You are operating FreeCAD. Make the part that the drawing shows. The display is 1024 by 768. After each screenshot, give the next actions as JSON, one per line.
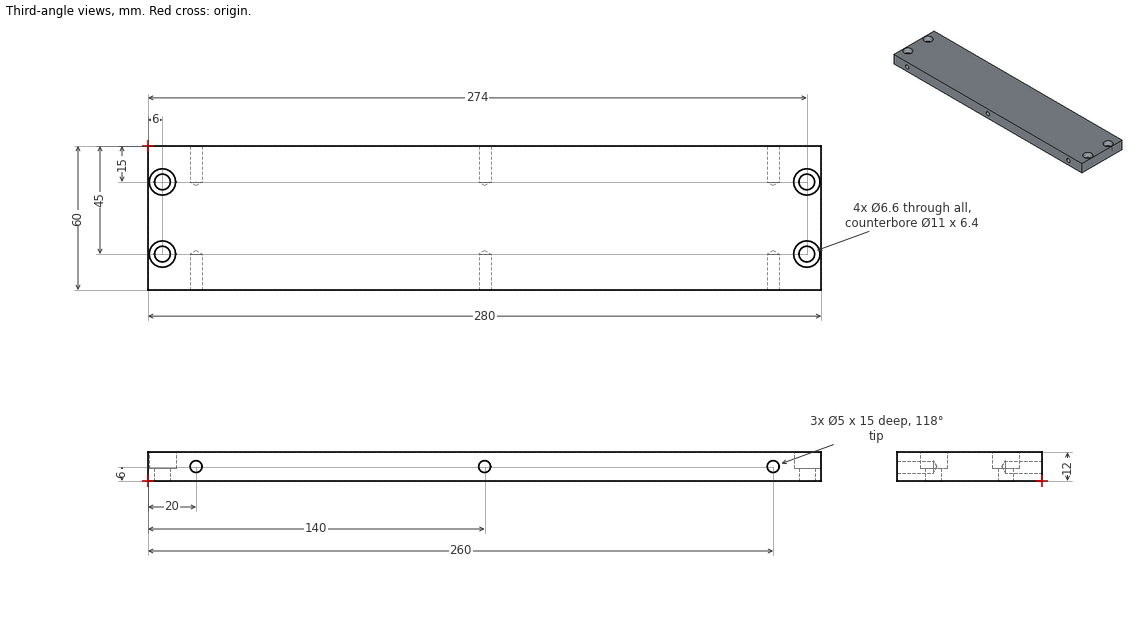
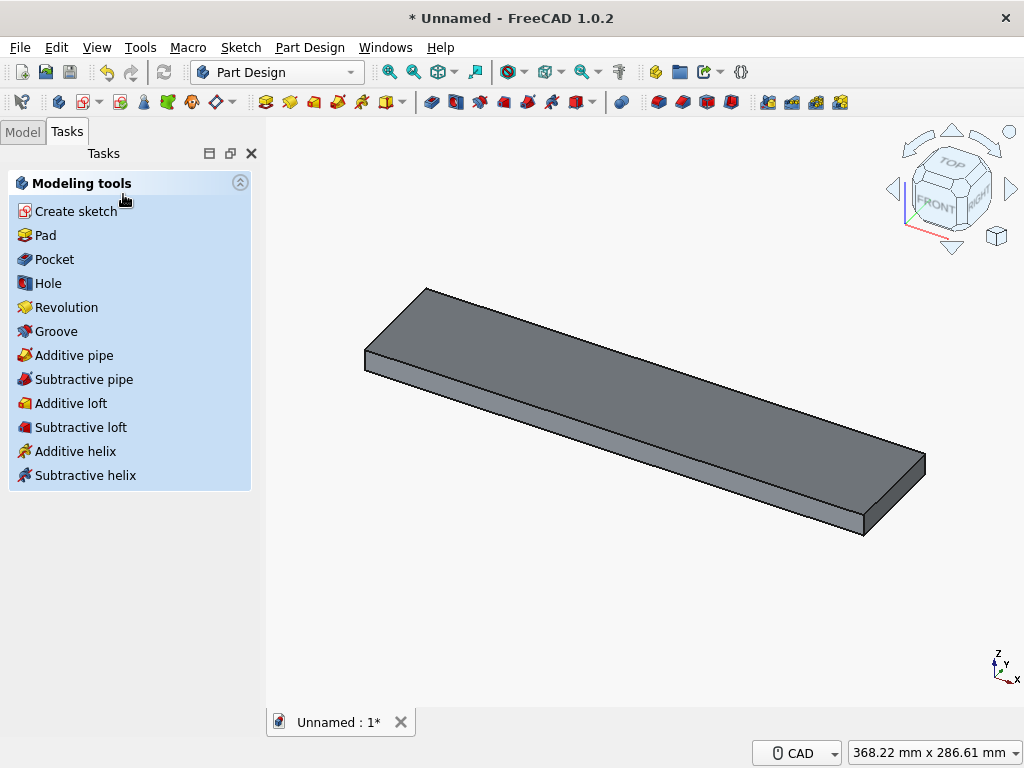
{"action": "left_click", "coordinate": [456, 102]}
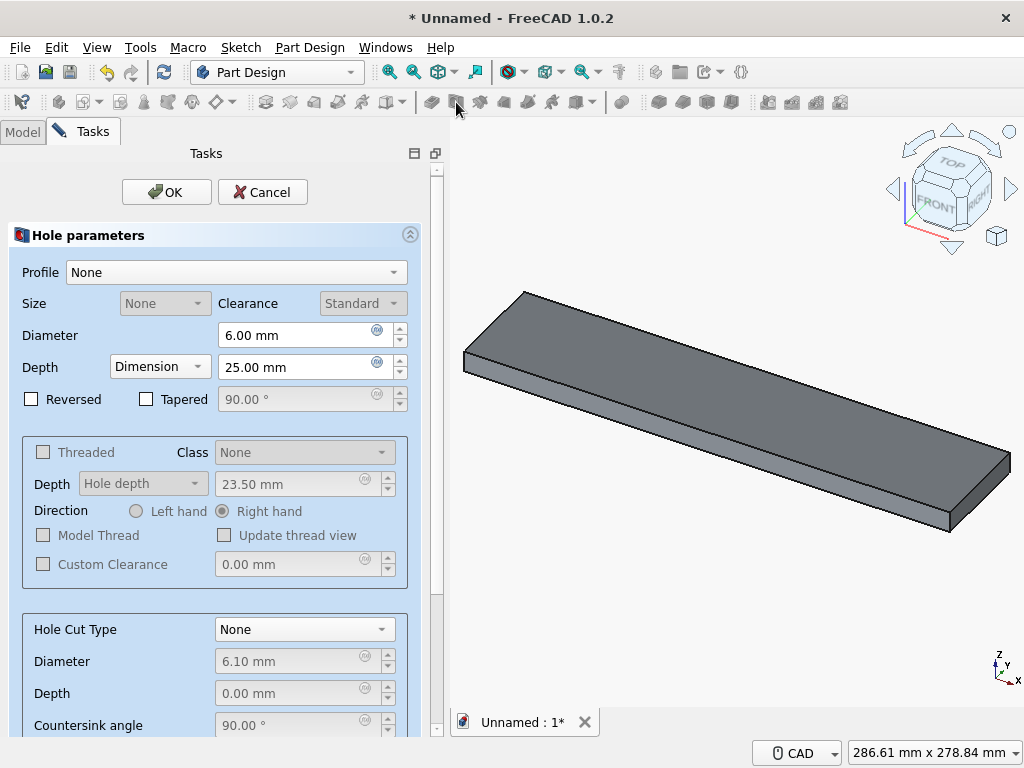
{"action": "triple_click", "coordinate": [305, 335]}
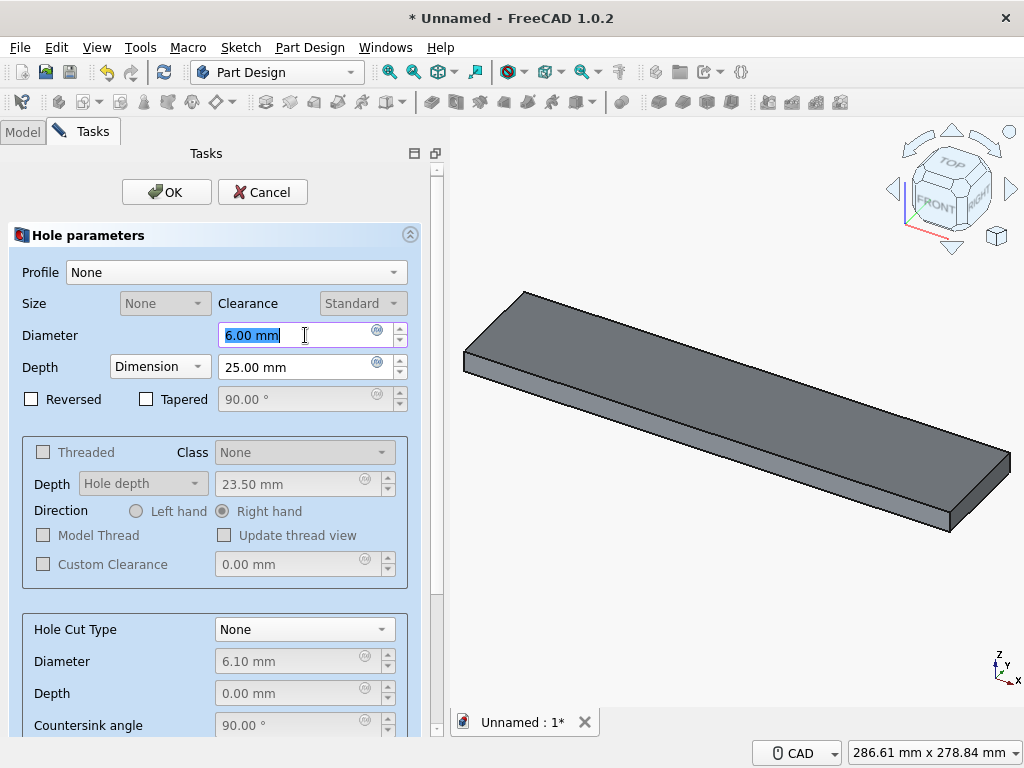
{"action": "type", "text": "5"}
{"action": "key", "text": "Tab"}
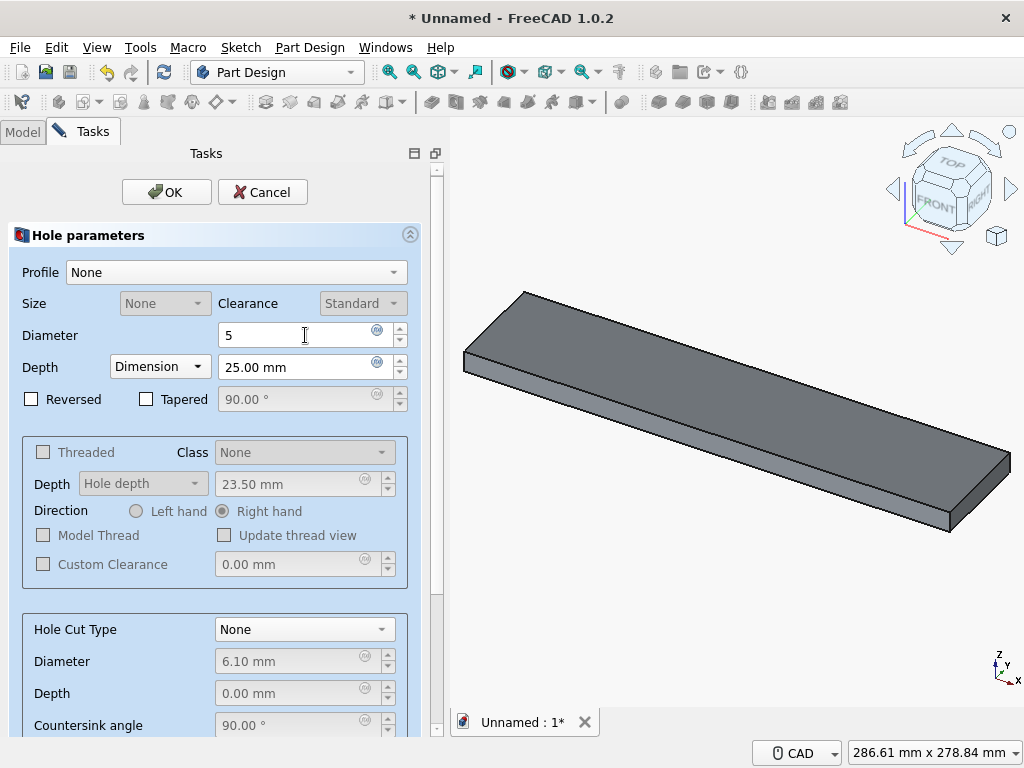
{"action": "triple_click", "coordinate": [305, 367]}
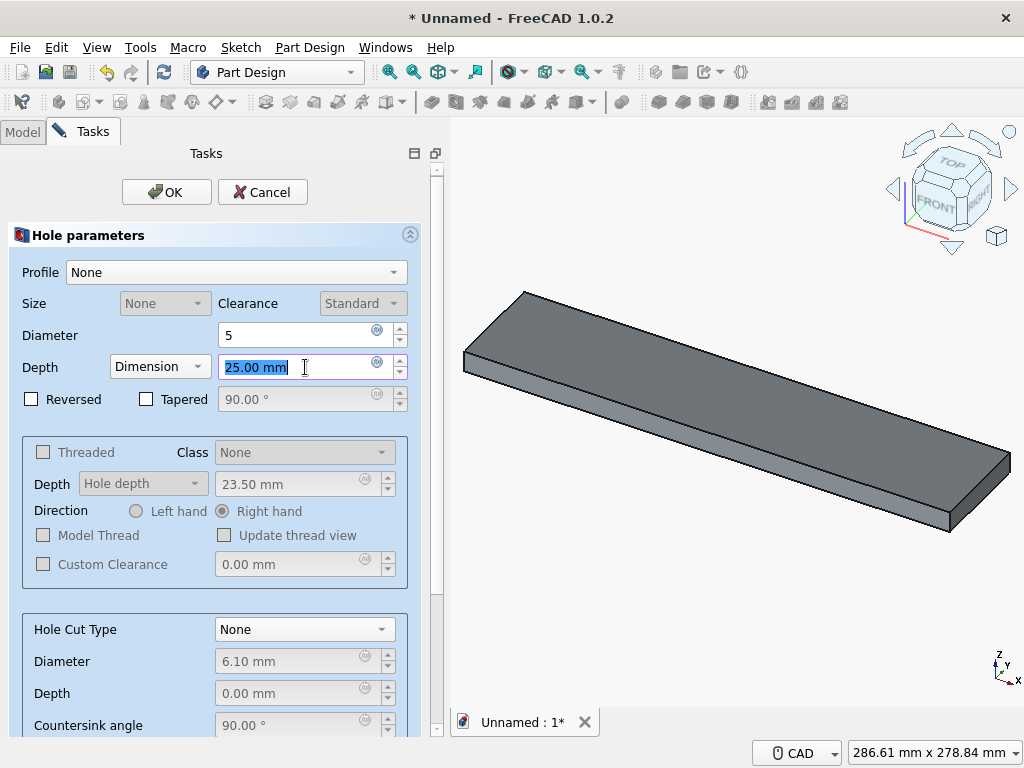
{"action": "type", "text": "15"}
{"action": "key", "text": "Tab"}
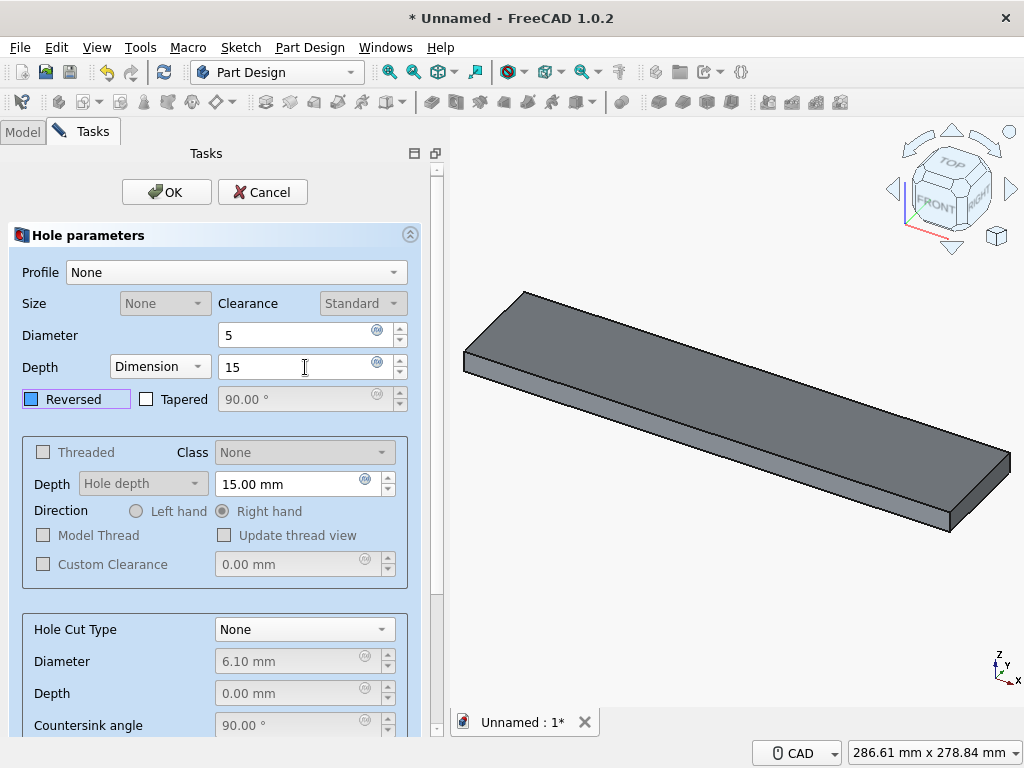
{"action": "left_click", "coordinate": [30, 399]}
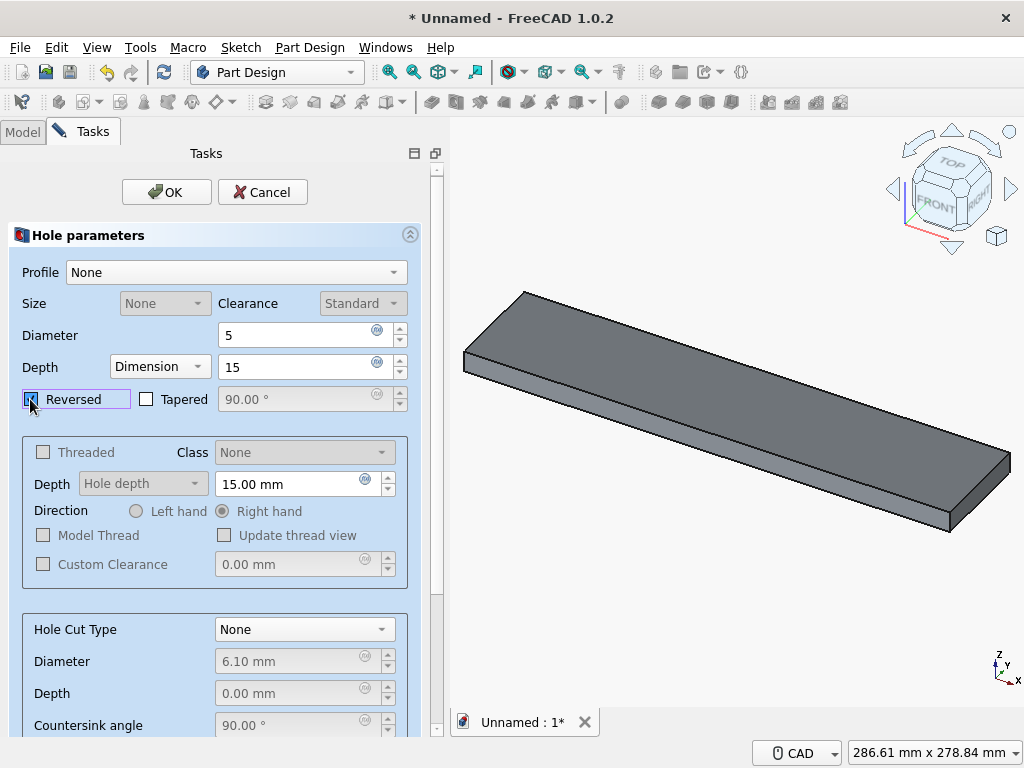
{"action": "left_click", "coordinate": [167, 192]}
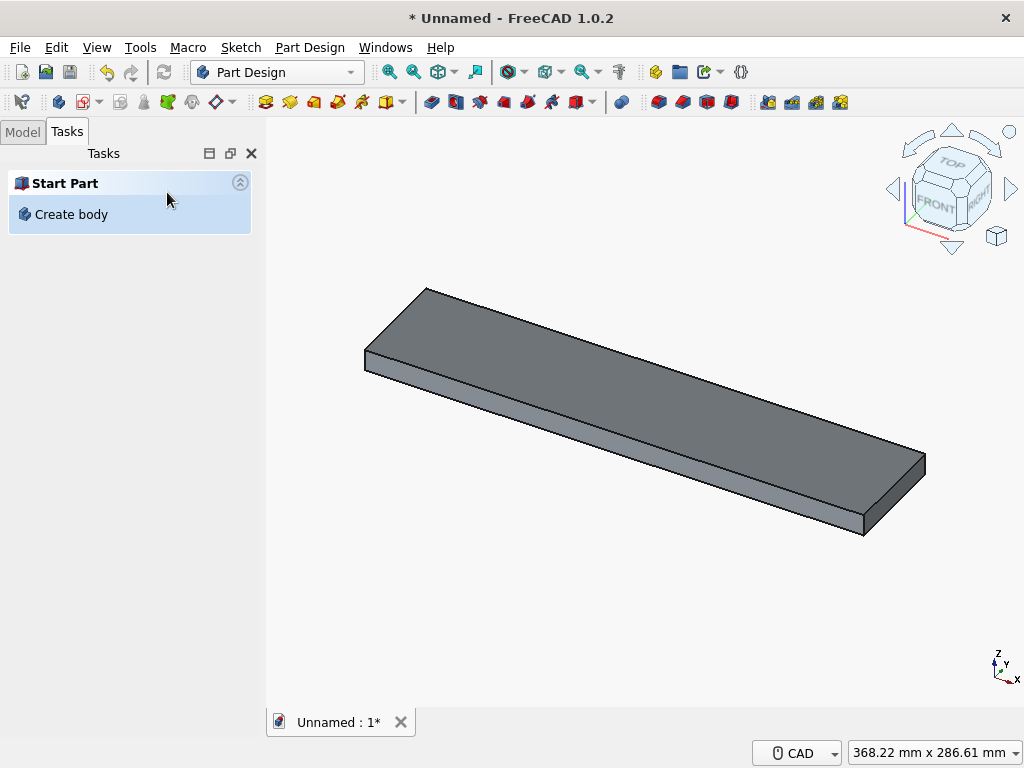
{"action": "left_click", "coordinate": [828, 513]}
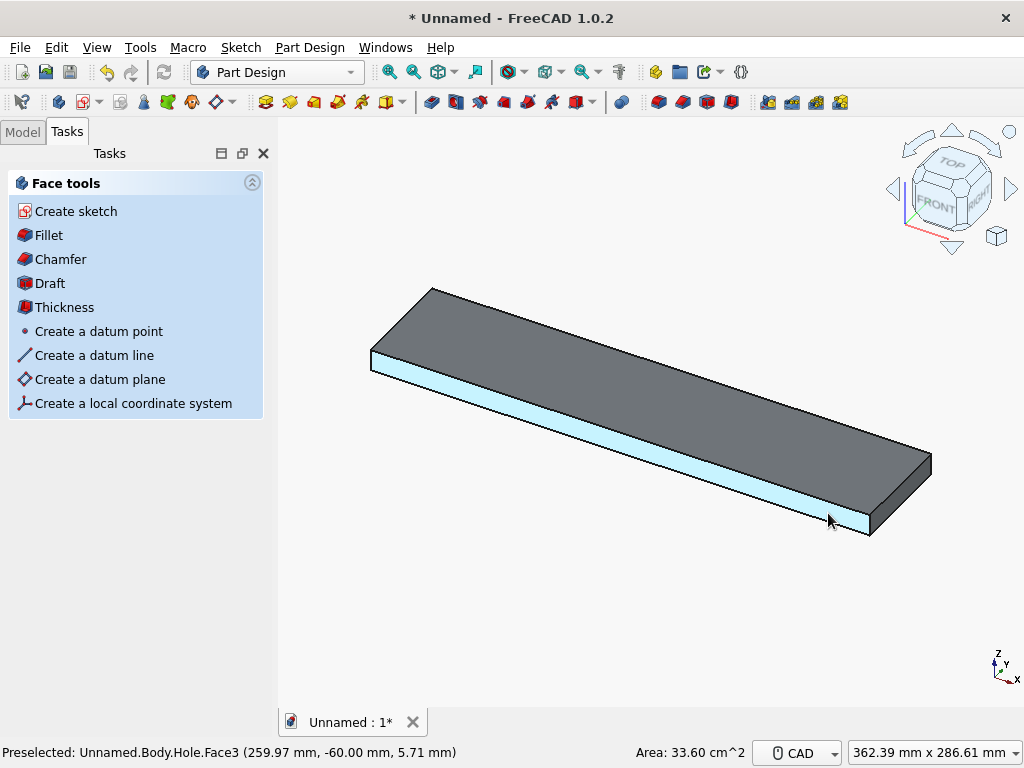
{"action": "left_click", "coordinate": [84, 102]}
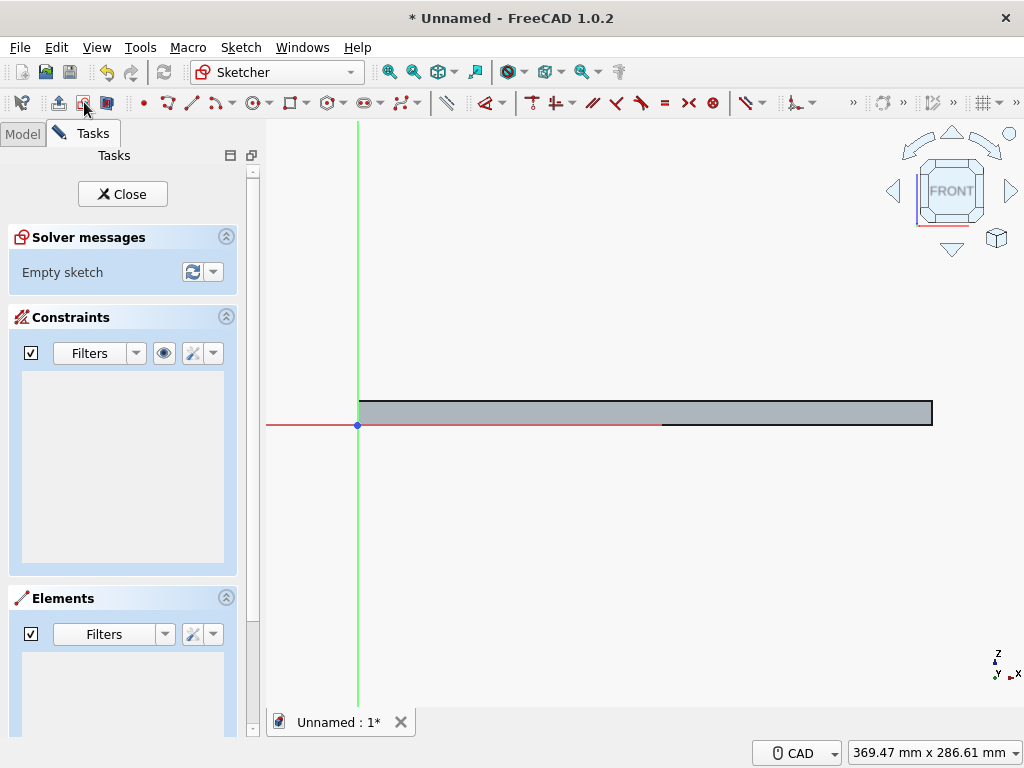
{"action": "scroll", "coordinate": [474, 406], "scroll_direction": "down", "scroll_amount": 2}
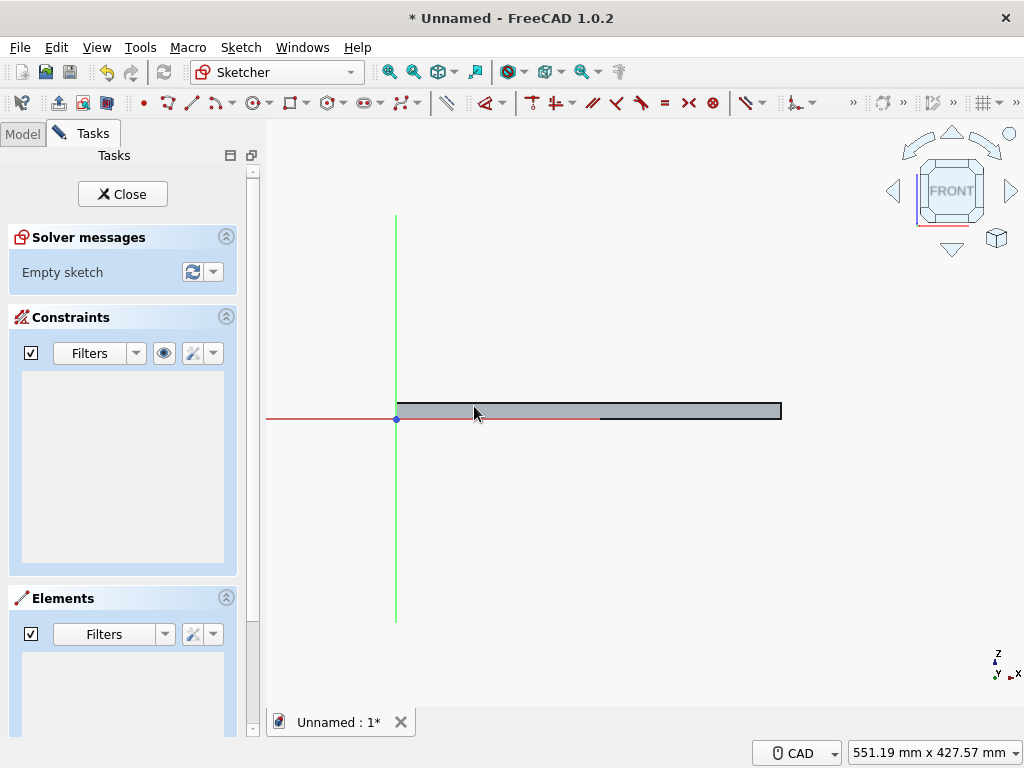
{"action": "left_click", "coordinate": [254, 104]}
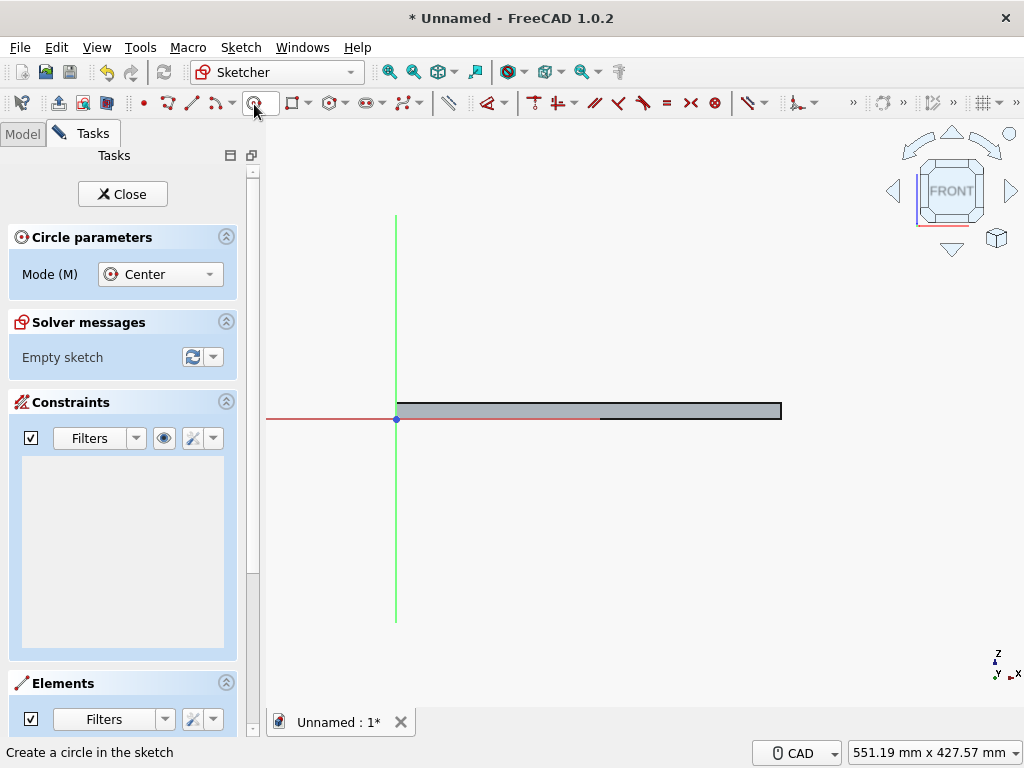
{"action": "scroll", "coordinate": [754, 411], "scroll_direction": "up", "scroll_amount": 10}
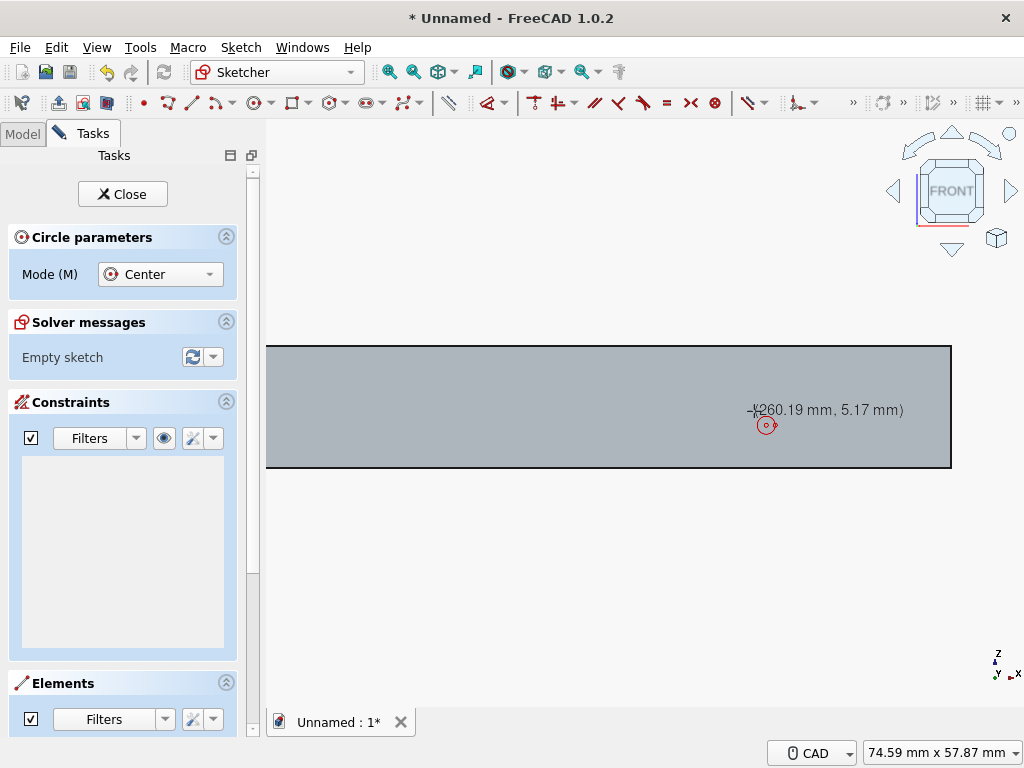
{"action": "scroll", "coordinate": [754, 411], "scroll_direction": "down", "scroll_amount": 10}